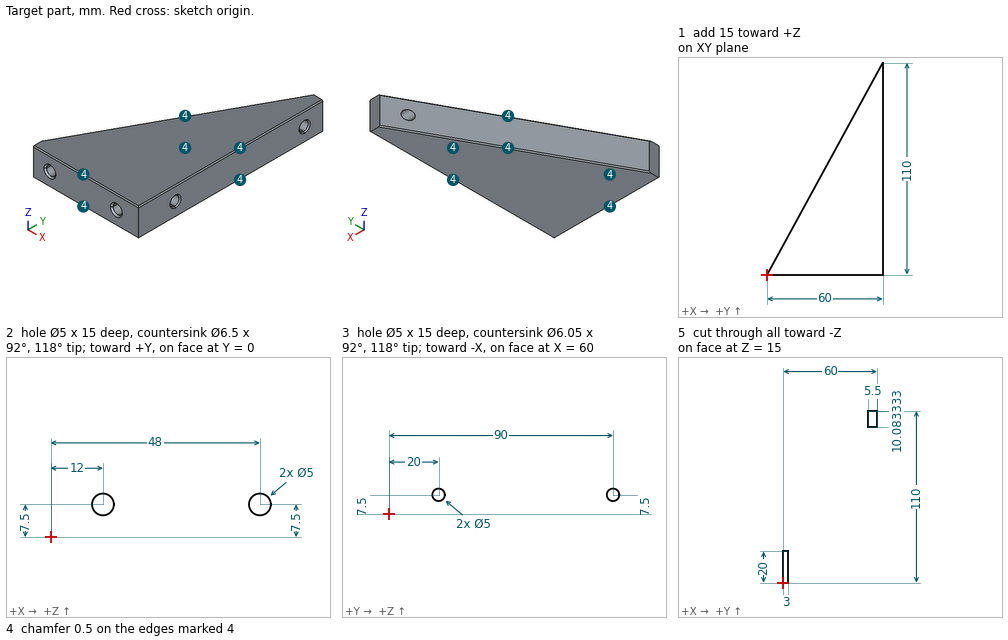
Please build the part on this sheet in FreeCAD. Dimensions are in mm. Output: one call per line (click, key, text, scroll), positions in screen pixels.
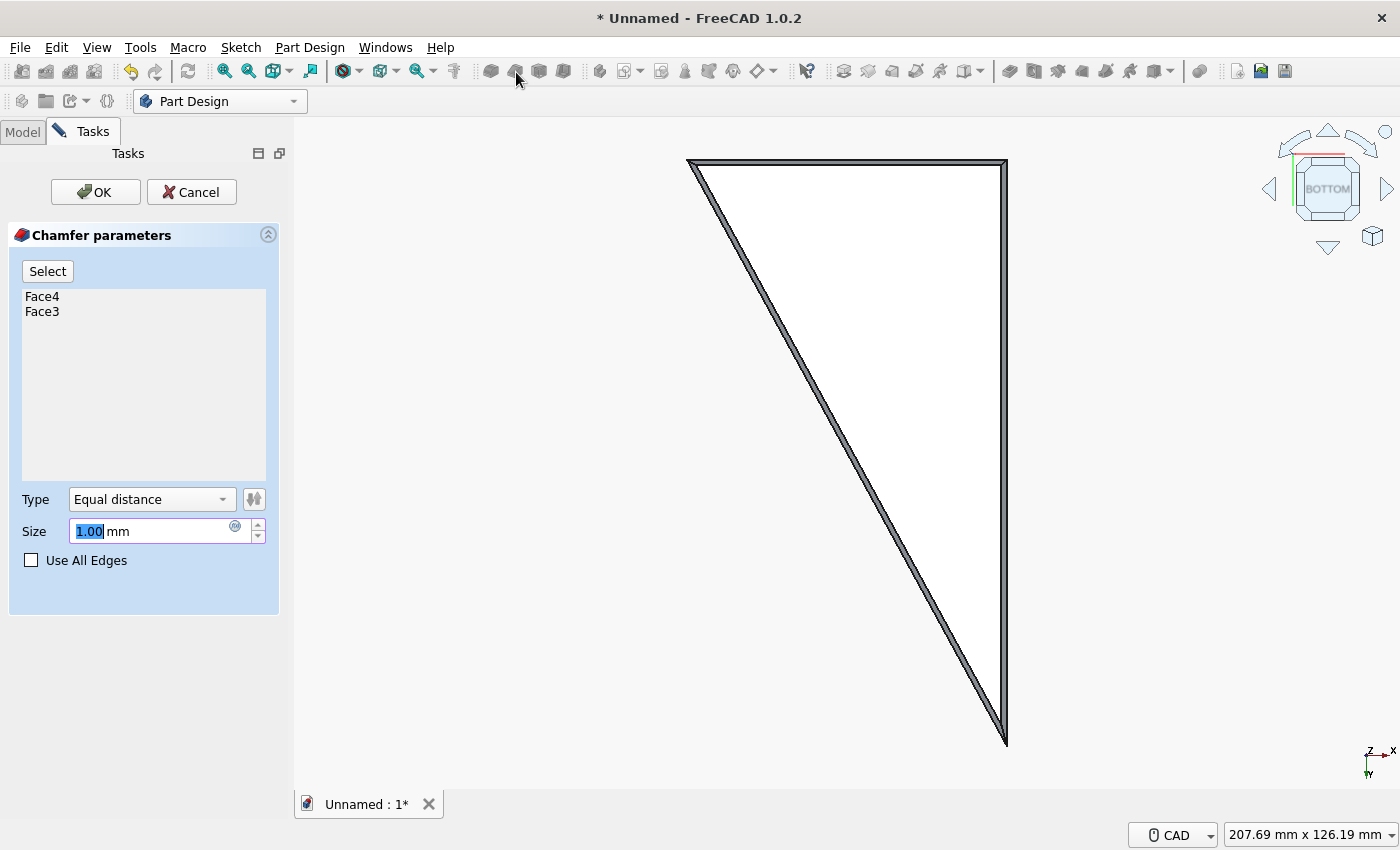
text(0.5)
key(Tab)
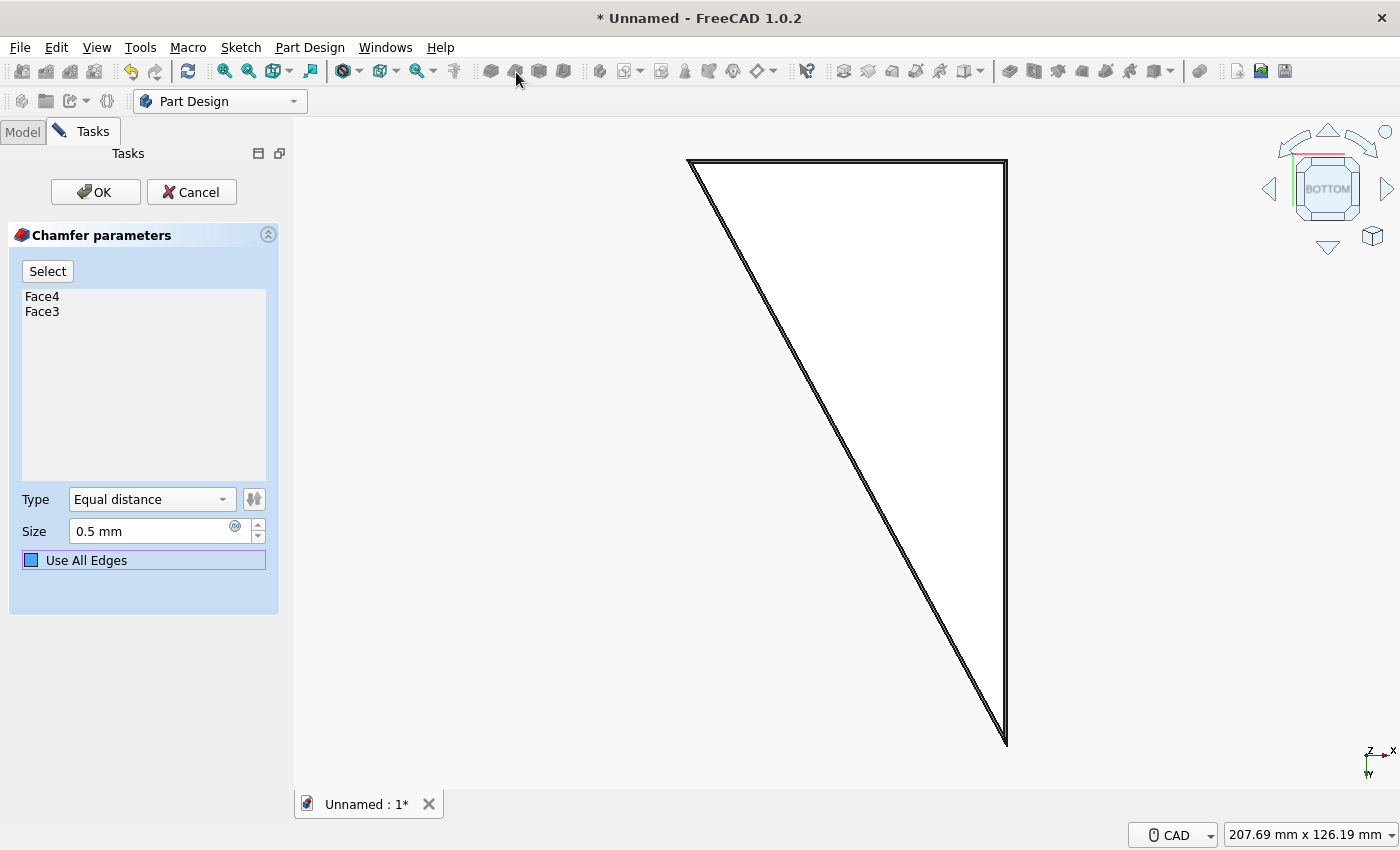
click(96, 192)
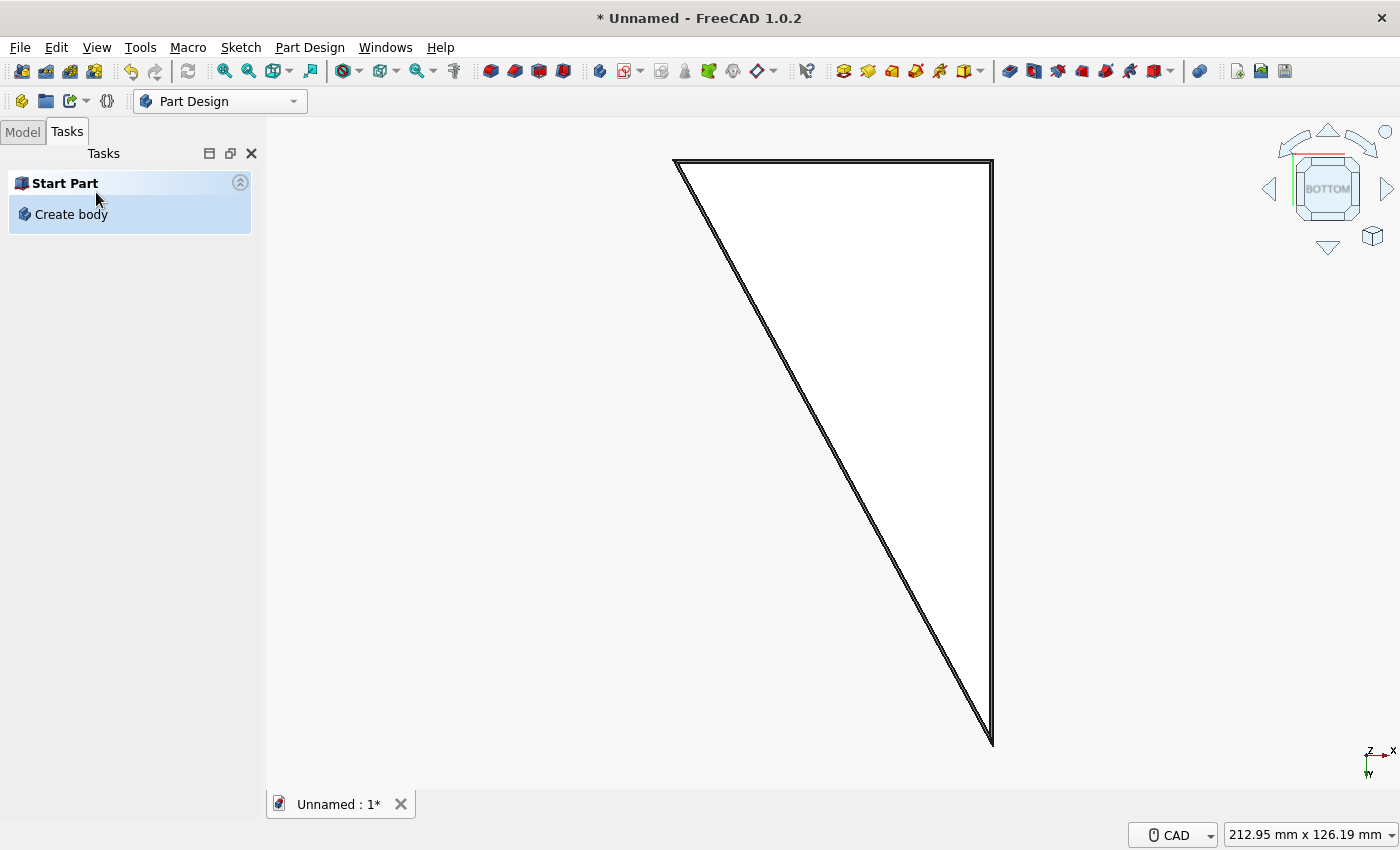
key(0)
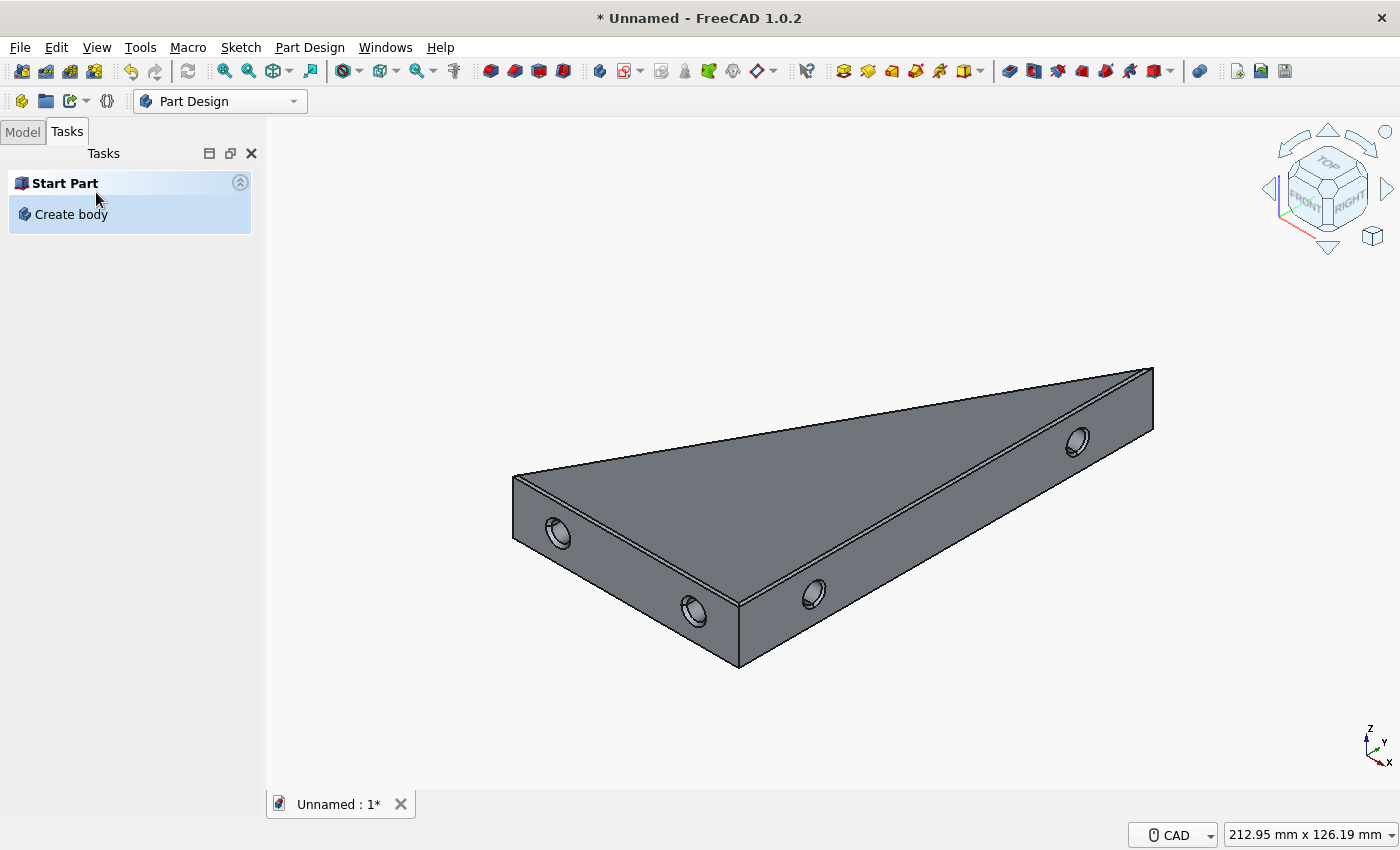
click(747, 506)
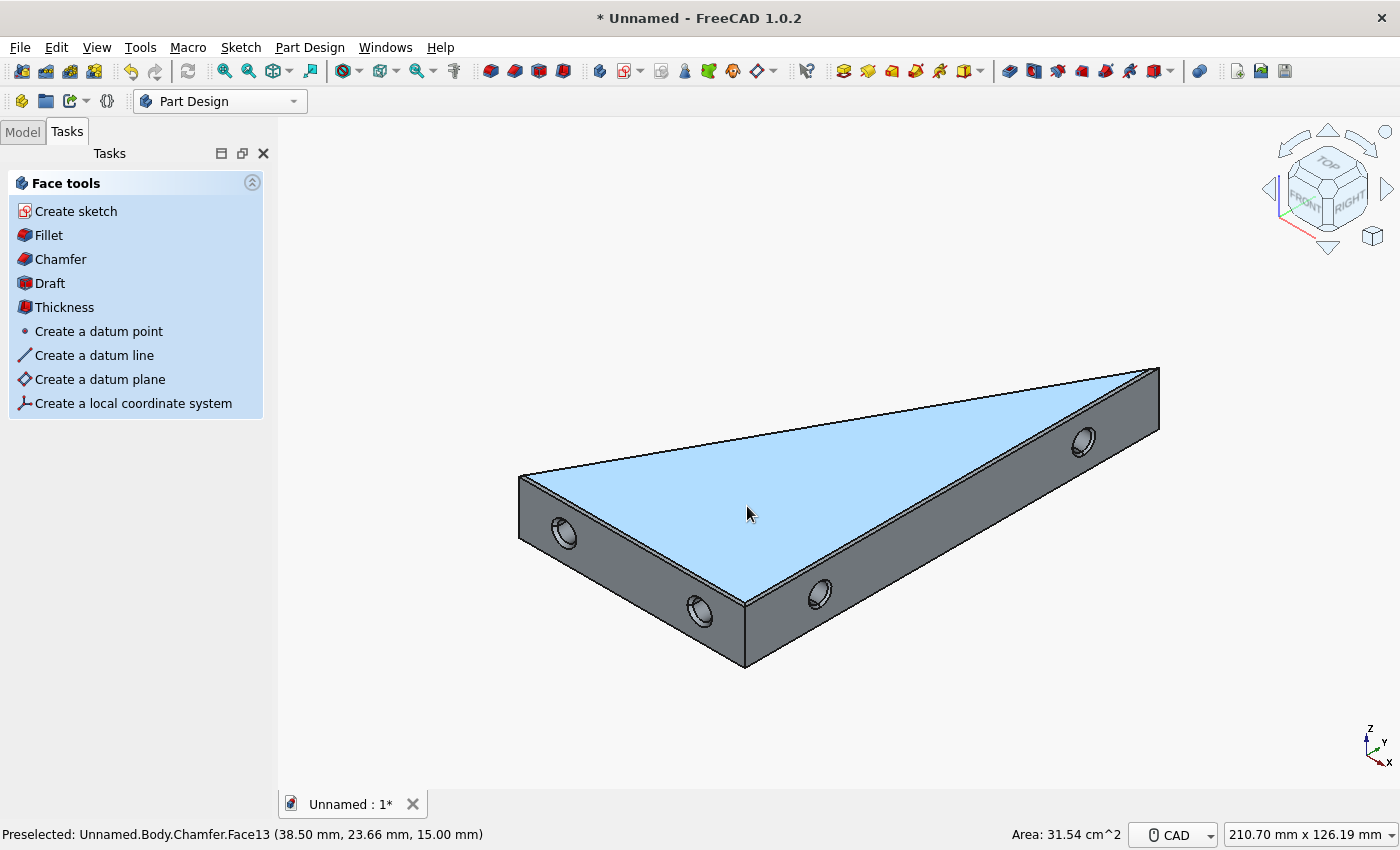
click(624, 72)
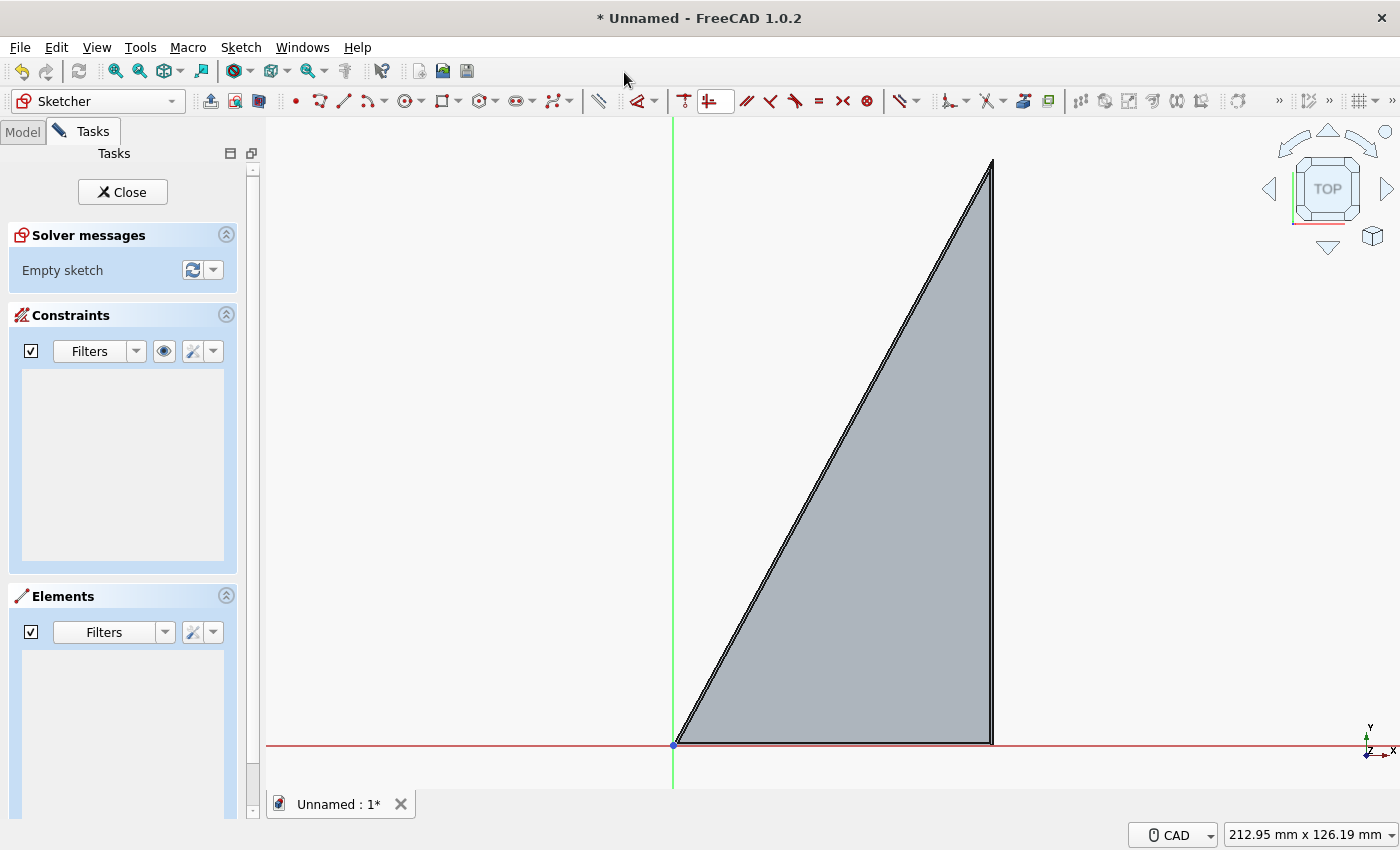
scroll(455, 453, down, 1)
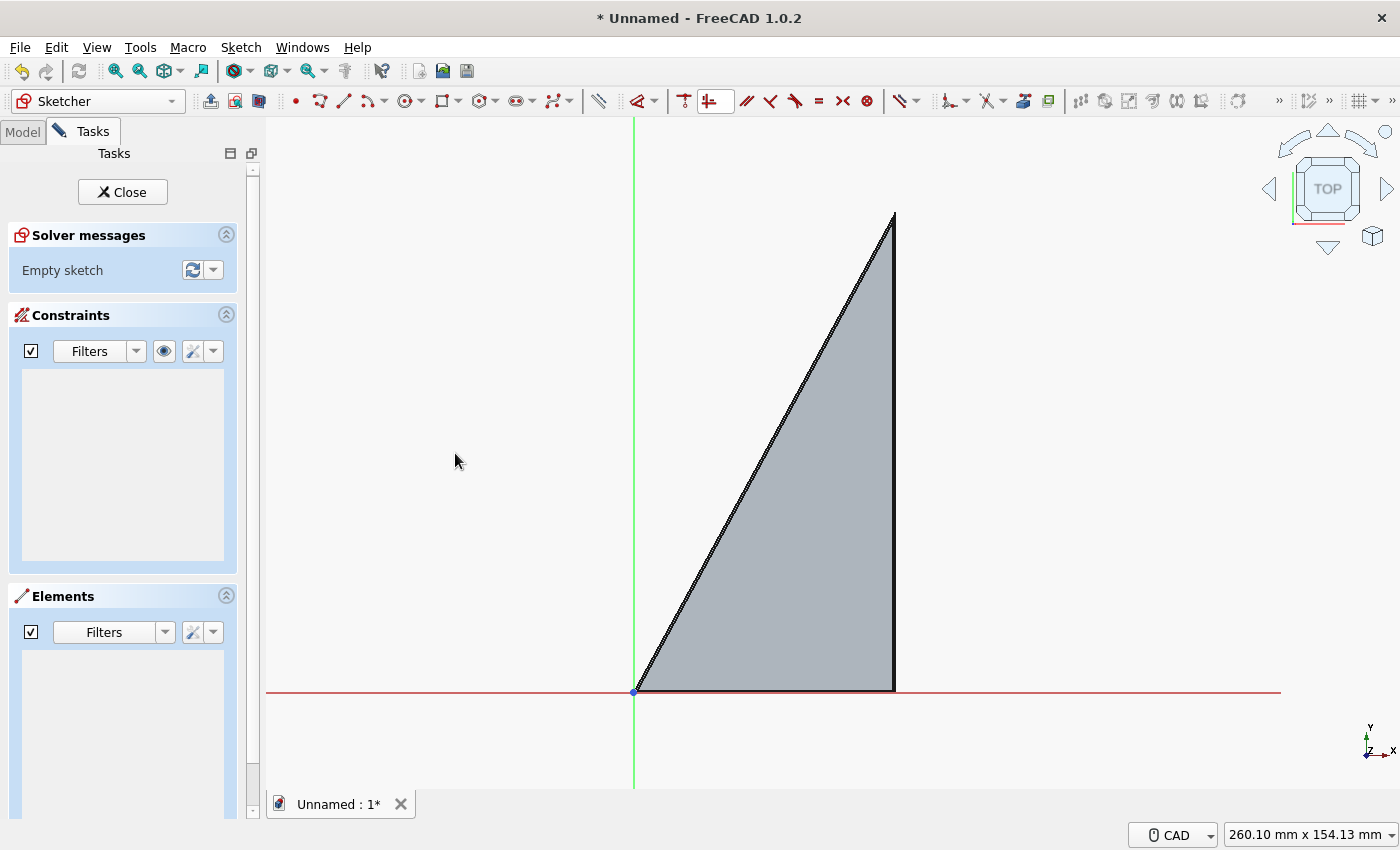
click(442, 102)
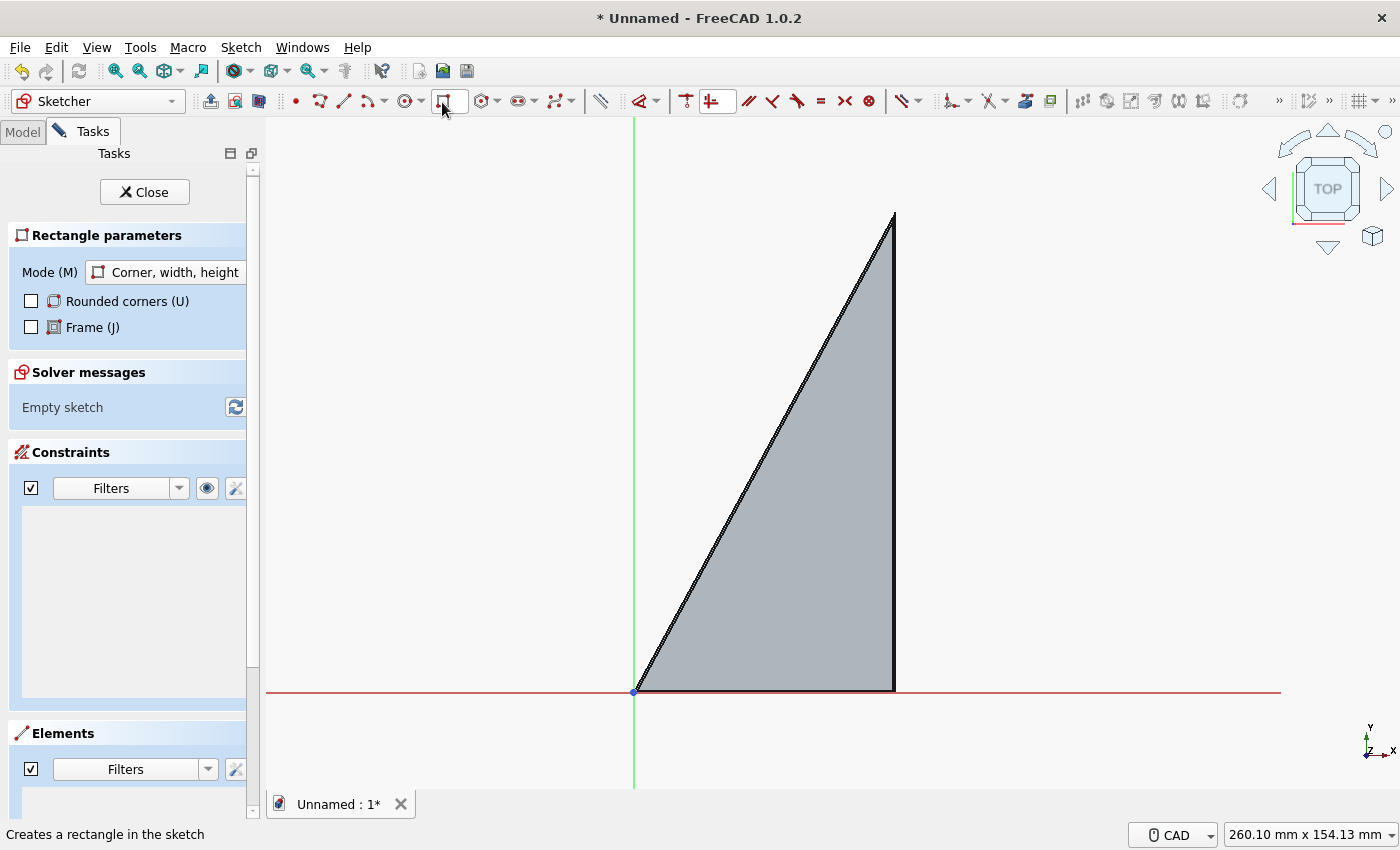
click(871, 213)
click(895, 257)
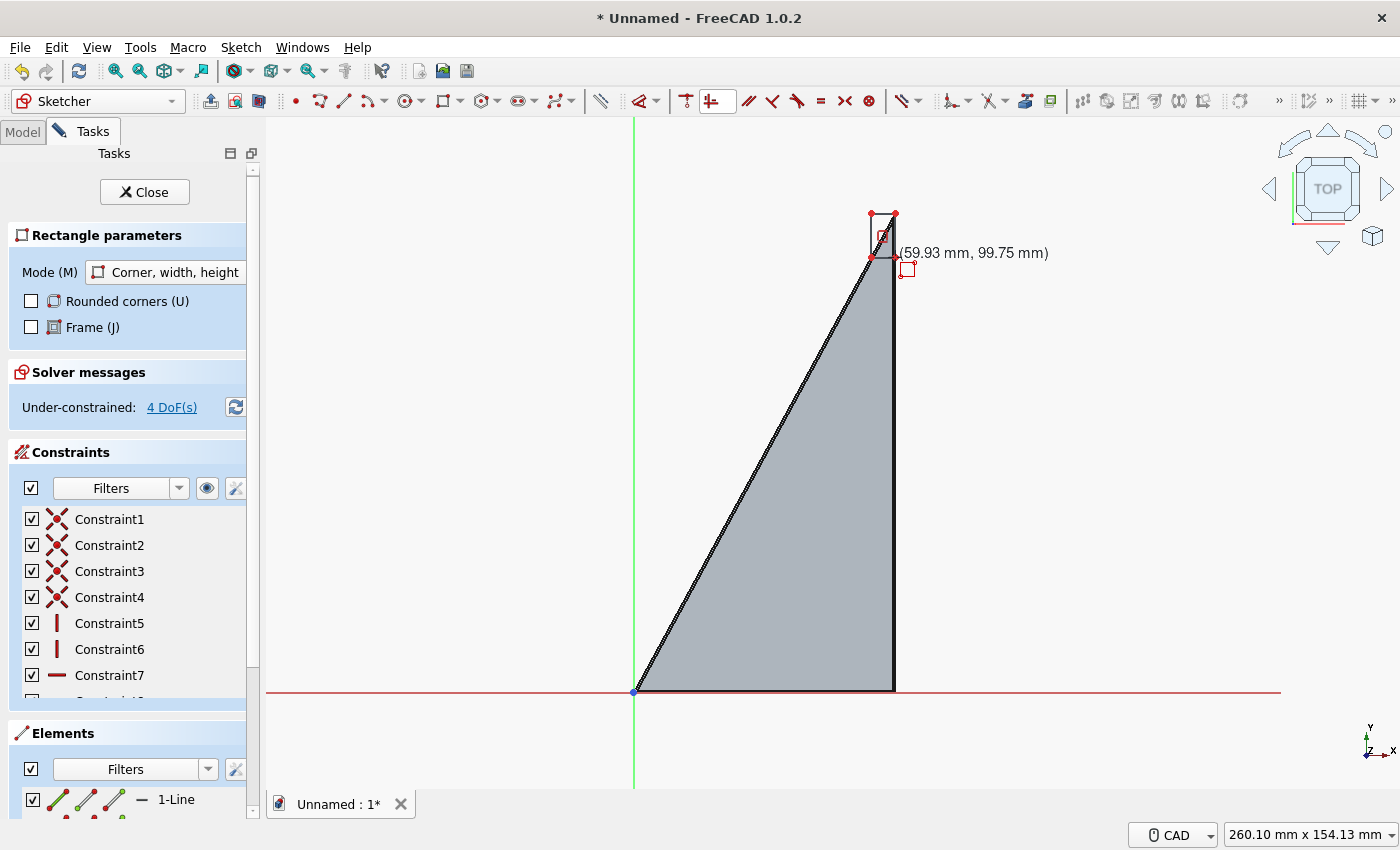
click(634, 693)
click(647, 606)
key(Escape)